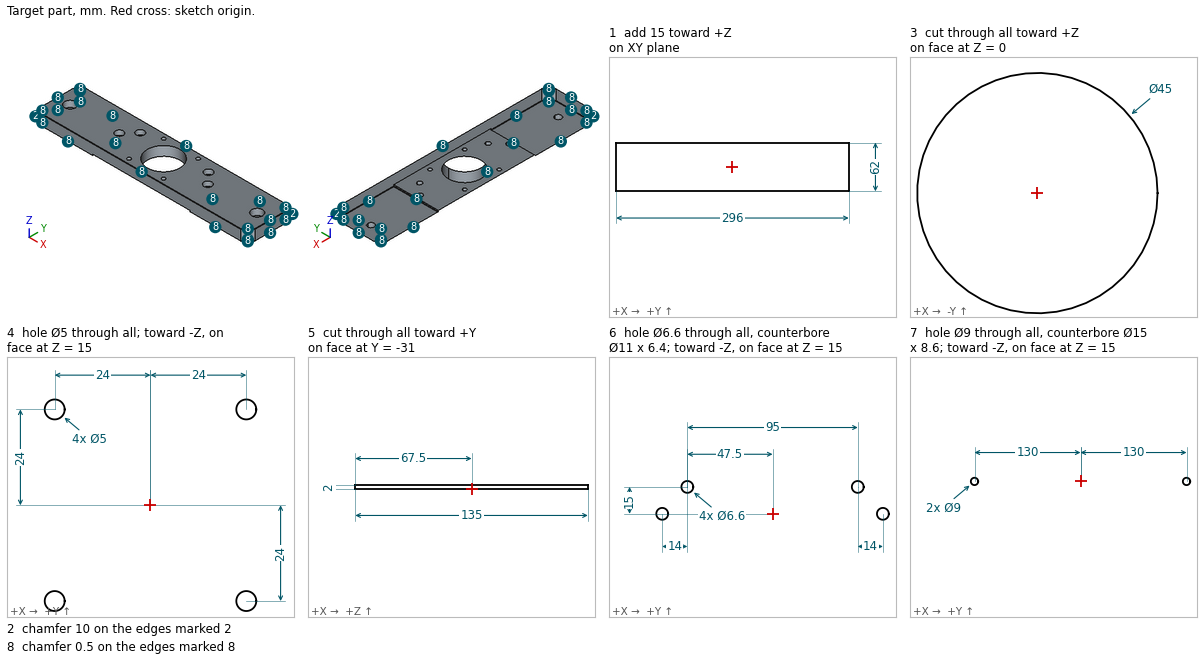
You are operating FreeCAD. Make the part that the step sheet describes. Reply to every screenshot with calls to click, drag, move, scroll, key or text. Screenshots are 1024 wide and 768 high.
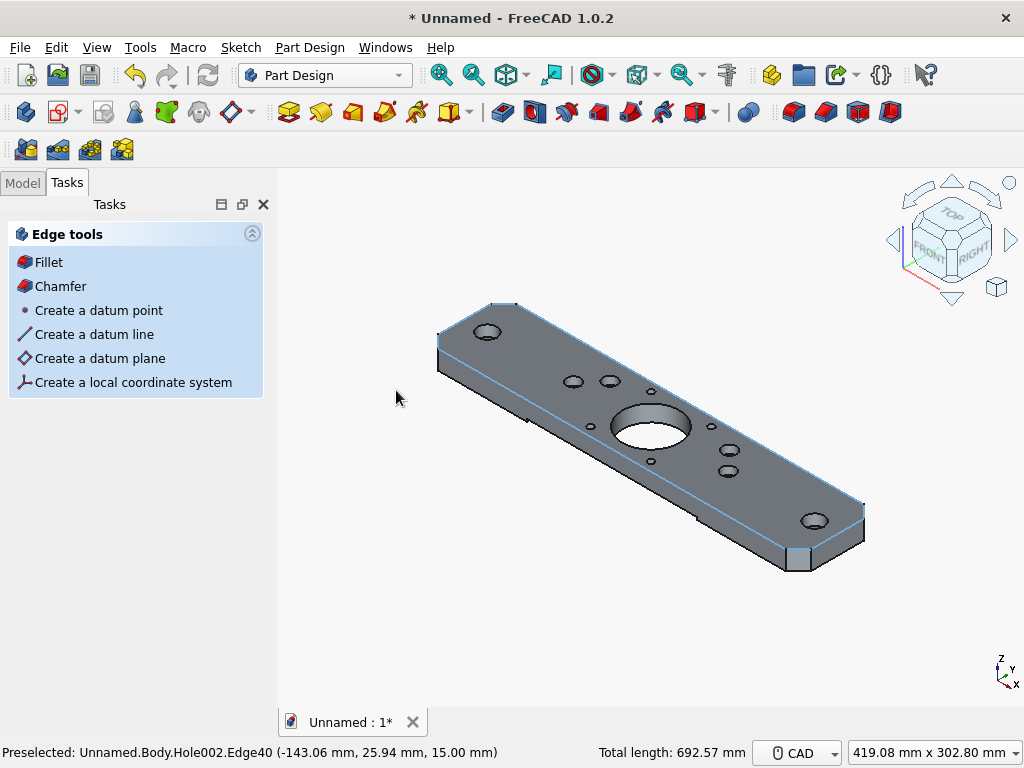
key(1)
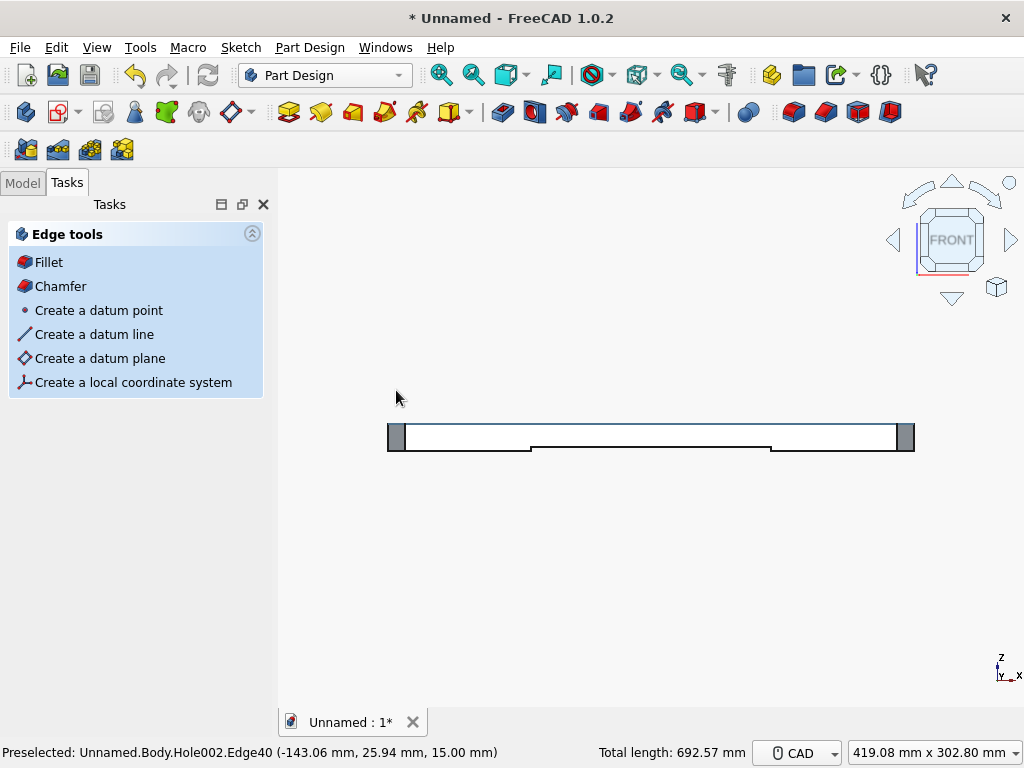
click(468, 450, ctrl)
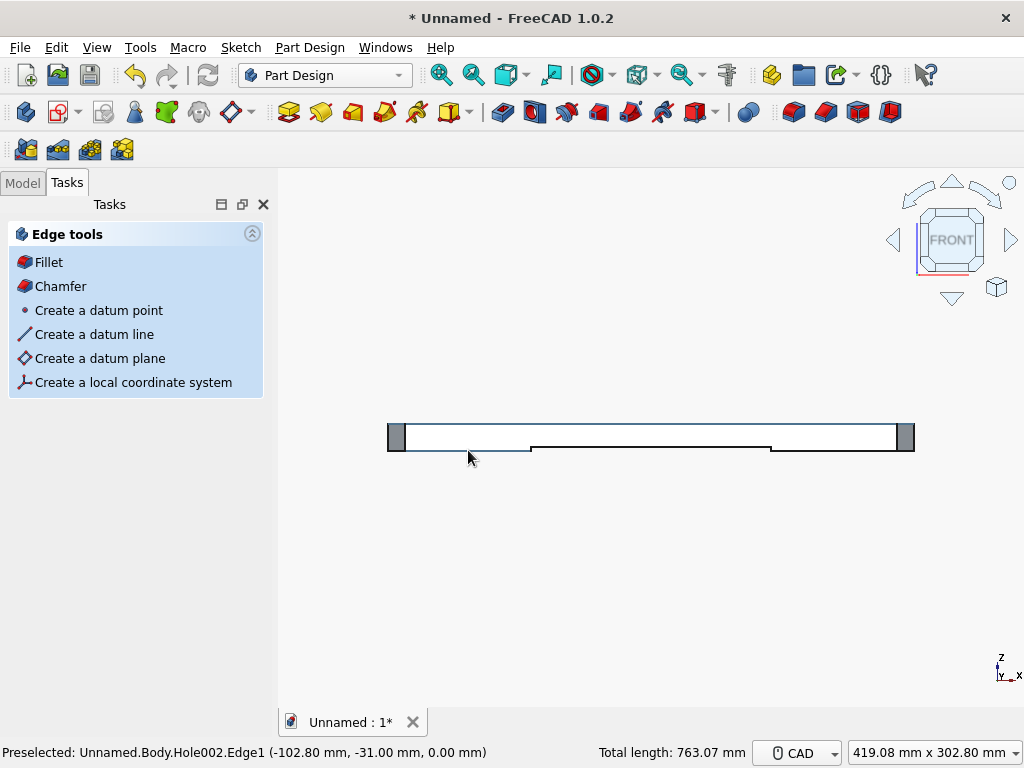
click(396, 450, ctrl)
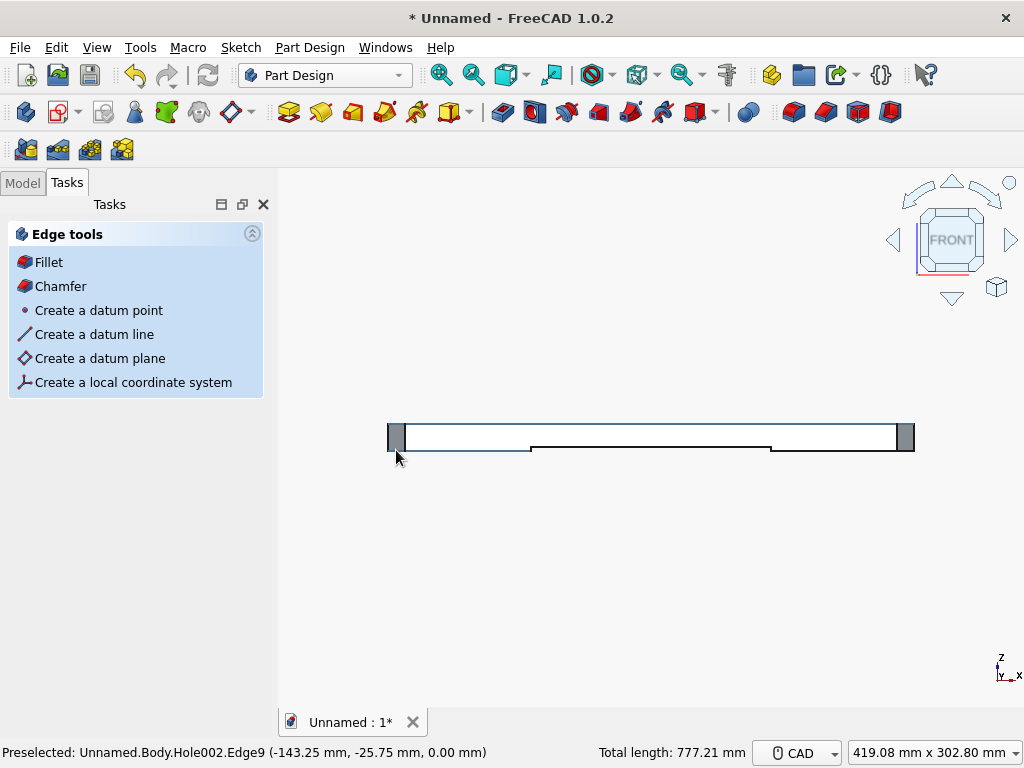
click(906, 450, ctrl)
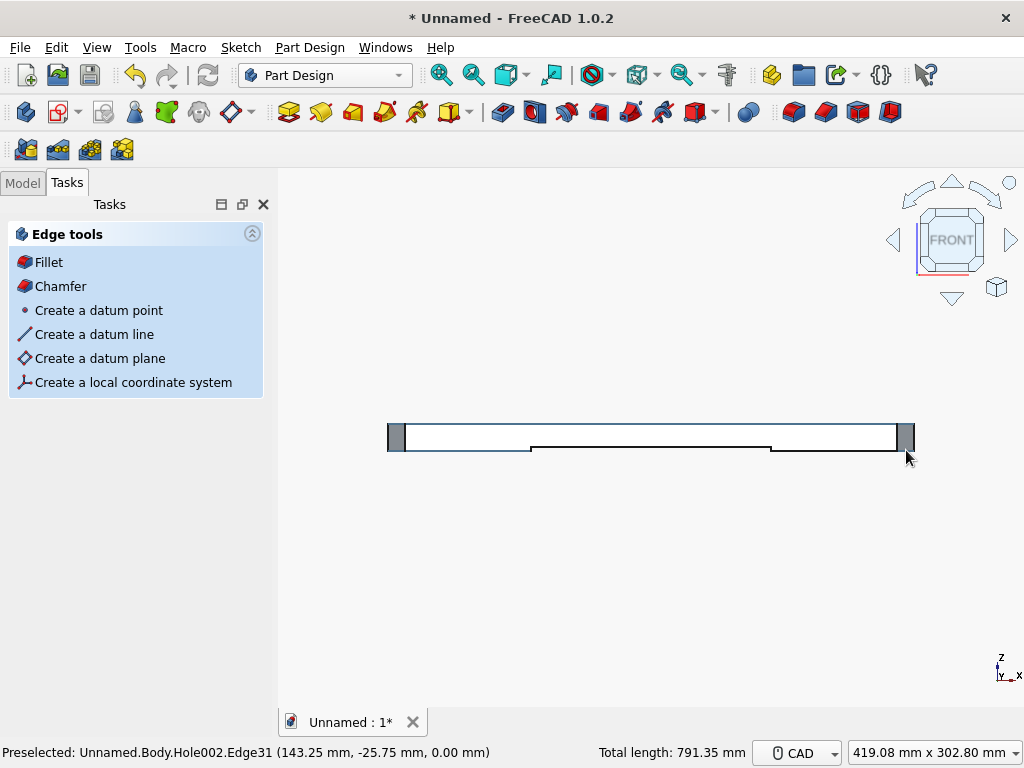
click(834, 450, ctrl)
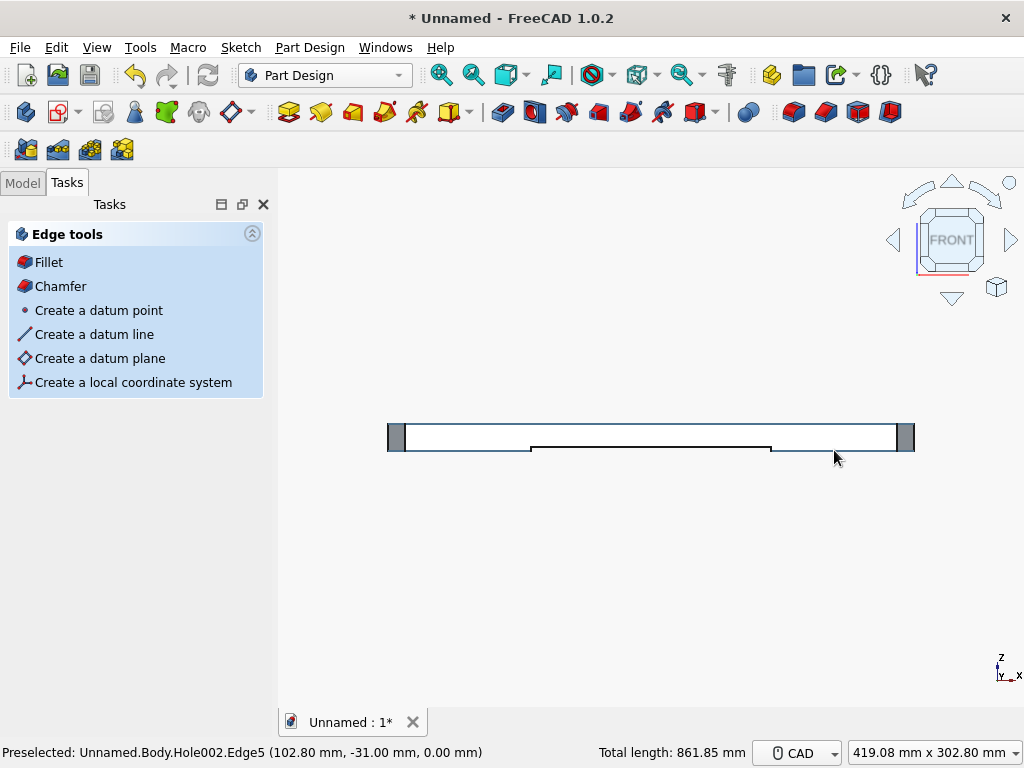
key(3)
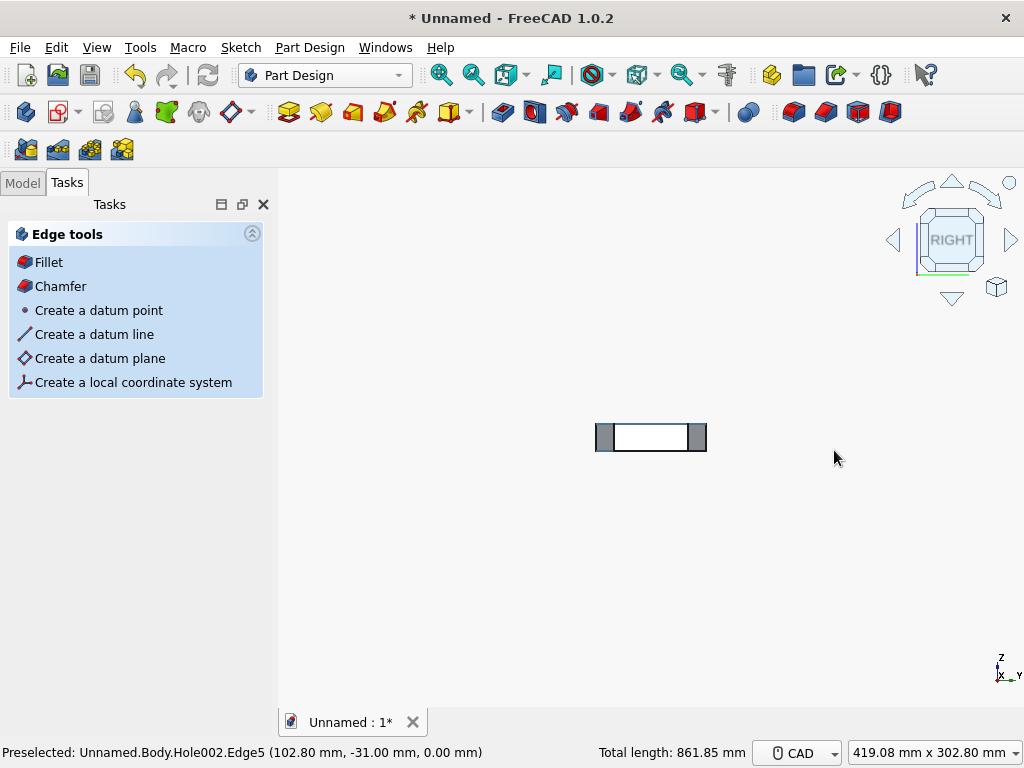
click(442, 76)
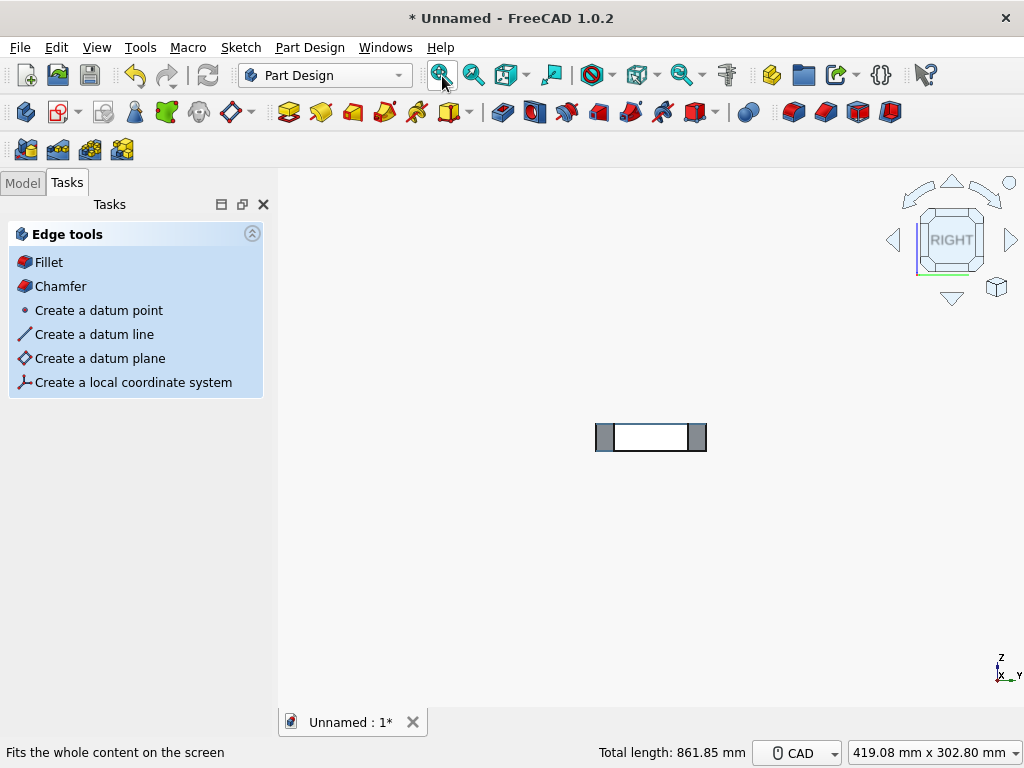
click(651, 450, ctrl)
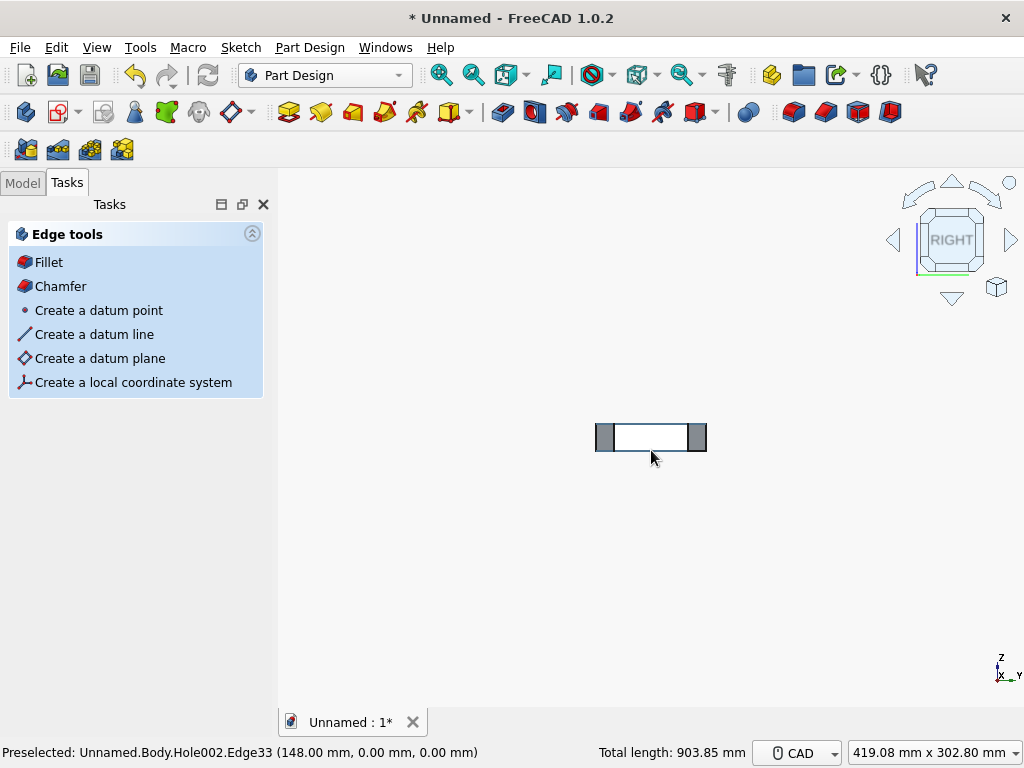
click(697, 450, ctrl)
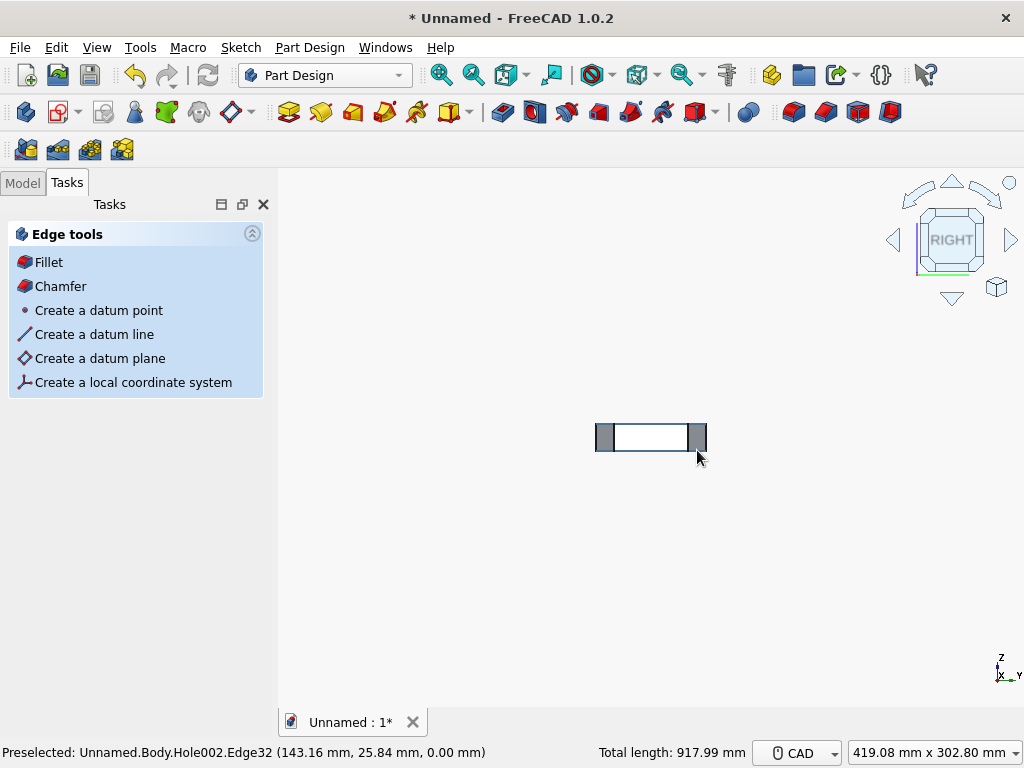
key(5)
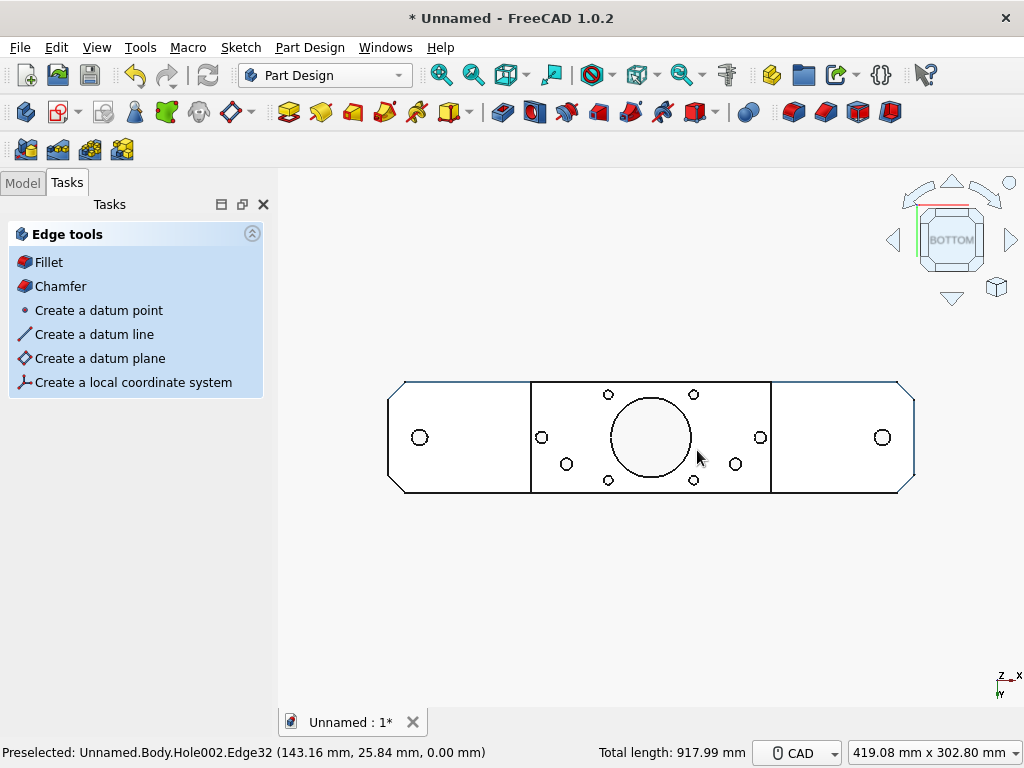
click(834, 492, ctrl)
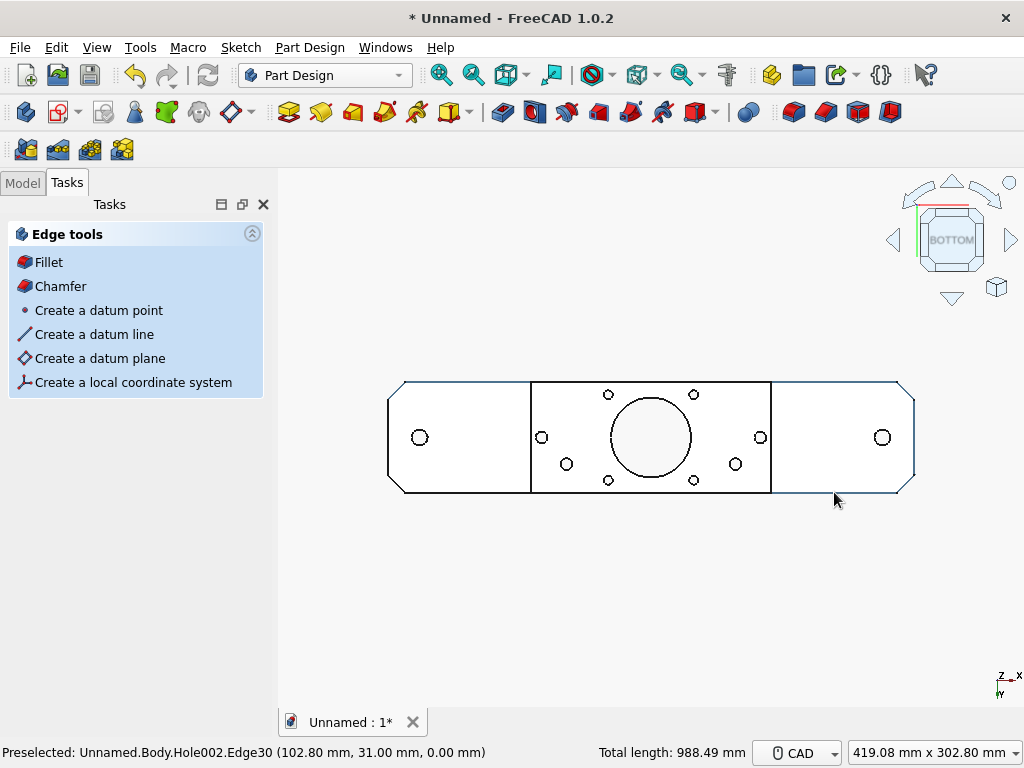
click(388, 436, ctrl)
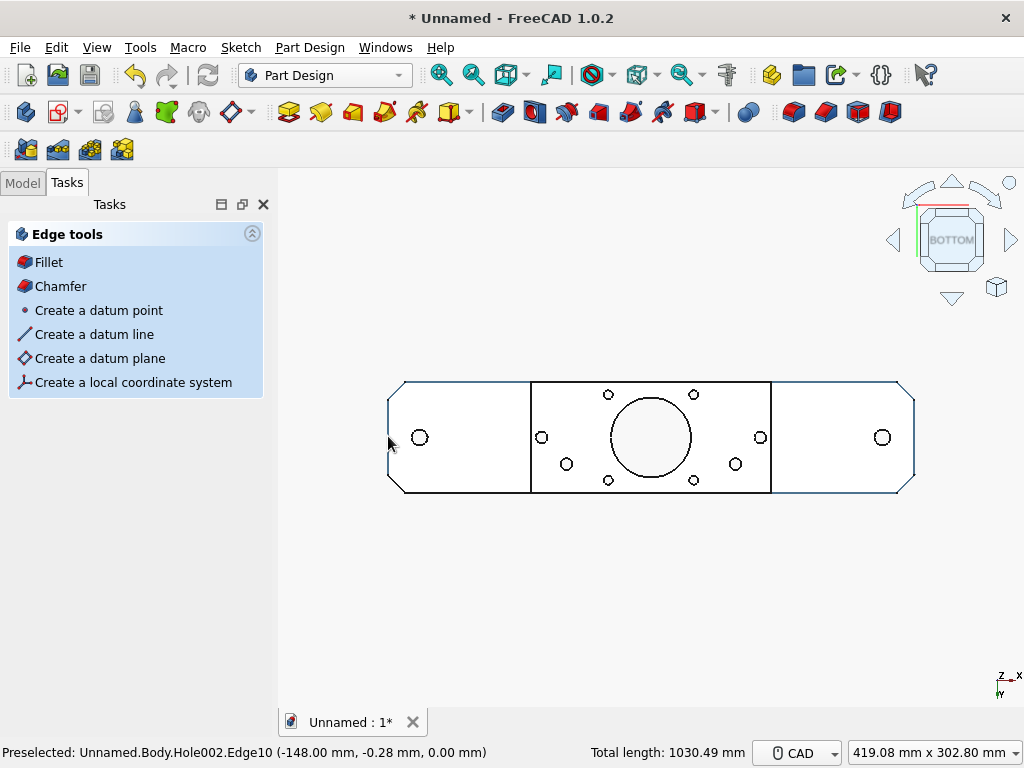
click(396, 483, ctrl)